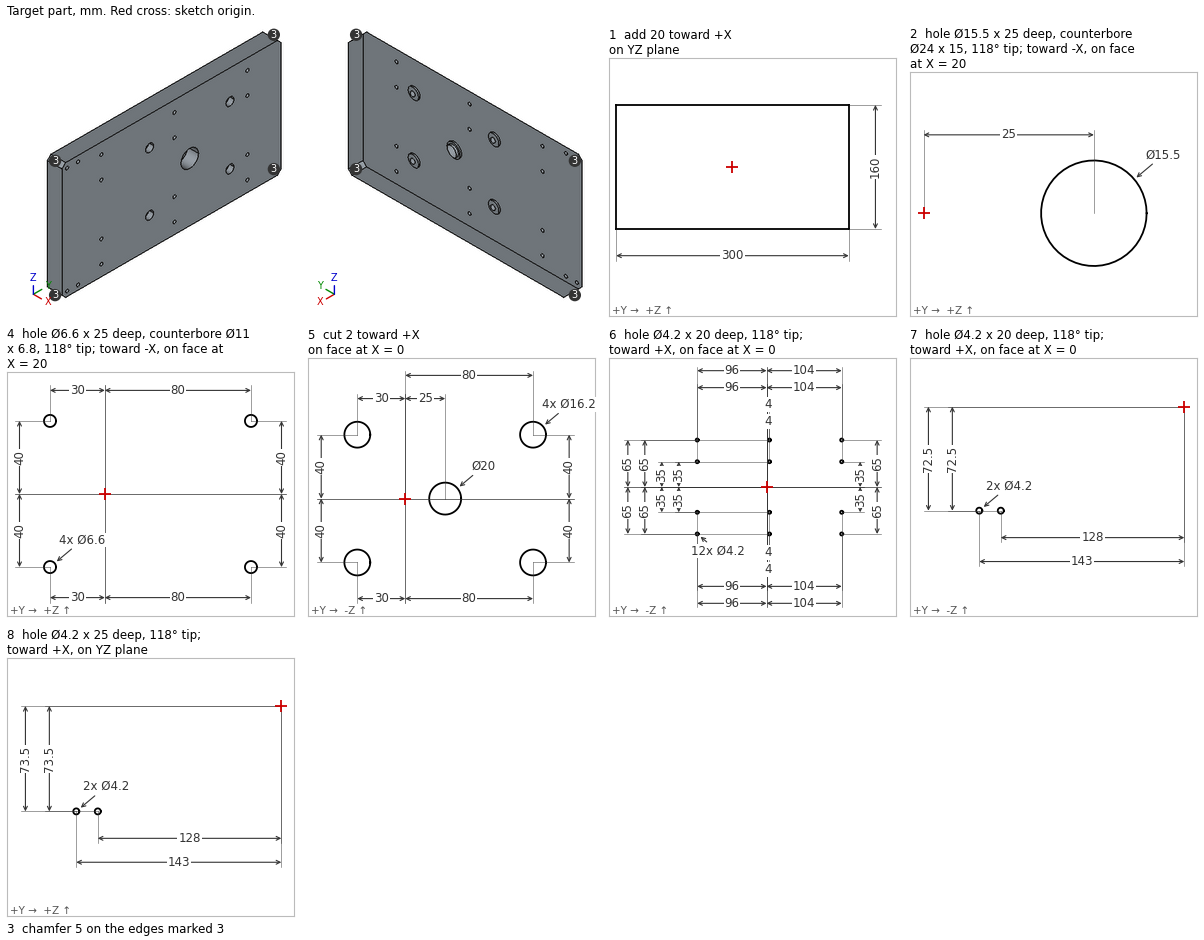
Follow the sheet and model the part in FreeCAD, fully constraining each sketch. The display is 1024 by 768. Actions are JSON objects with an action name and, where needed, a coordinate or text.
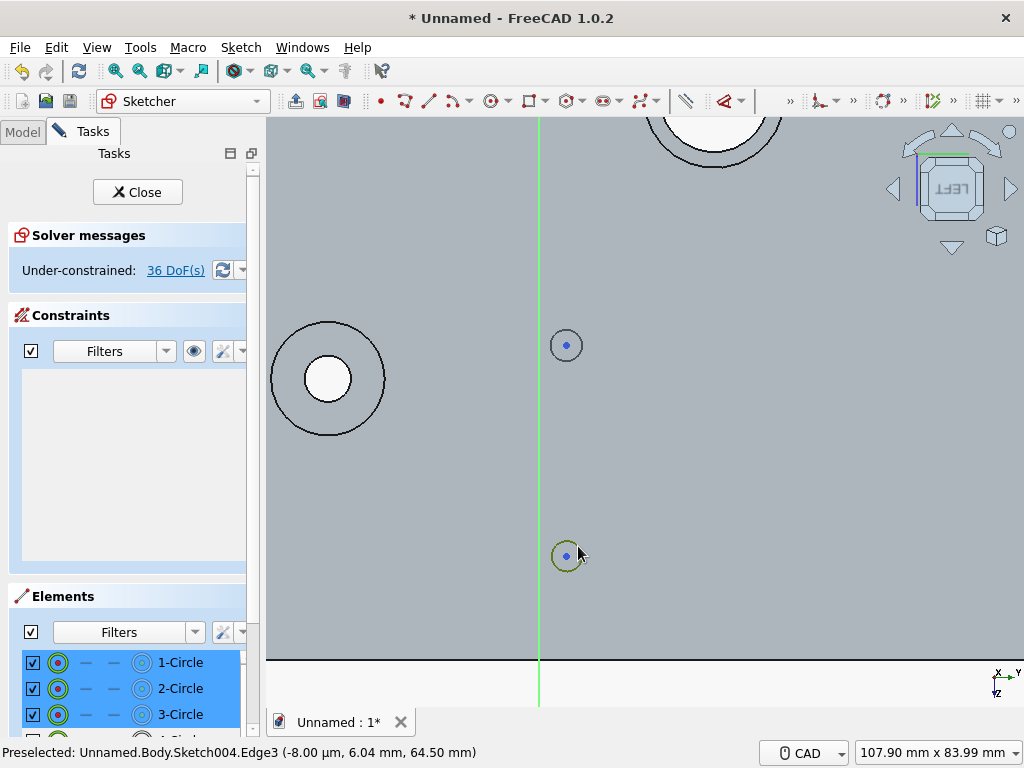
{"action": "left_click", "coordinate": [577, 334]}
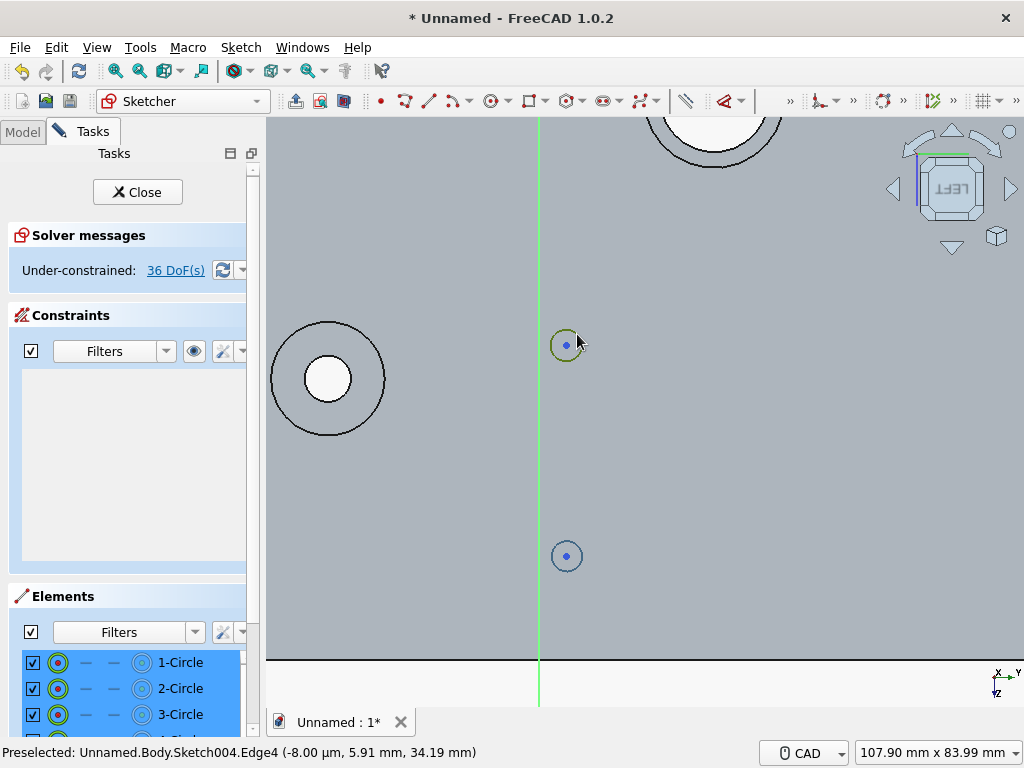
{"action": "scroll", "coordinate": [581, 547], "scroll_direction": "down", "scroll_amount": 6}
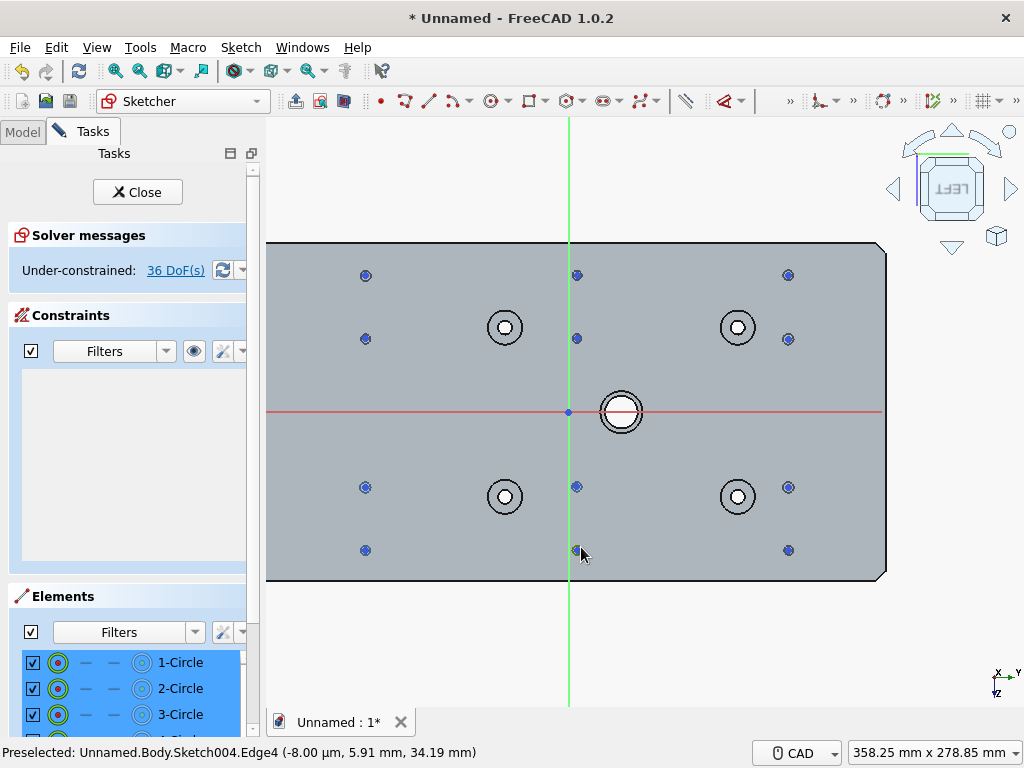
{"action": "scroll", "coordinate": [792, 547], "scroll_direction": "up", "scroll_amount": 6}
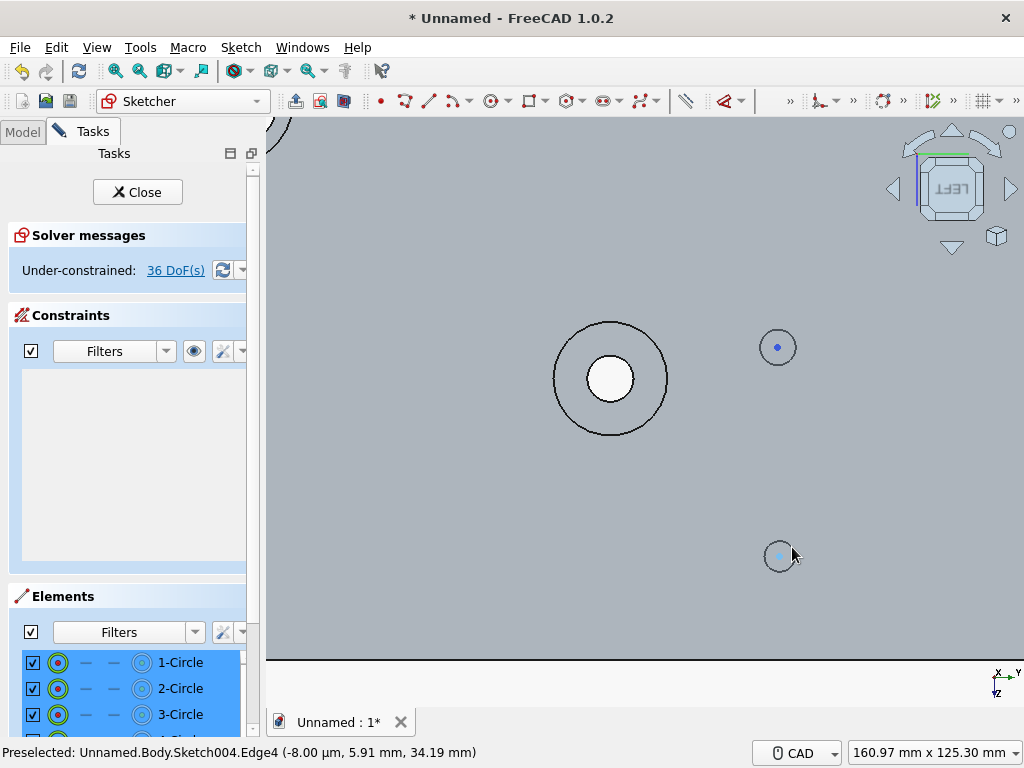
{"action": "left_click", "coordinate": [790, 546]}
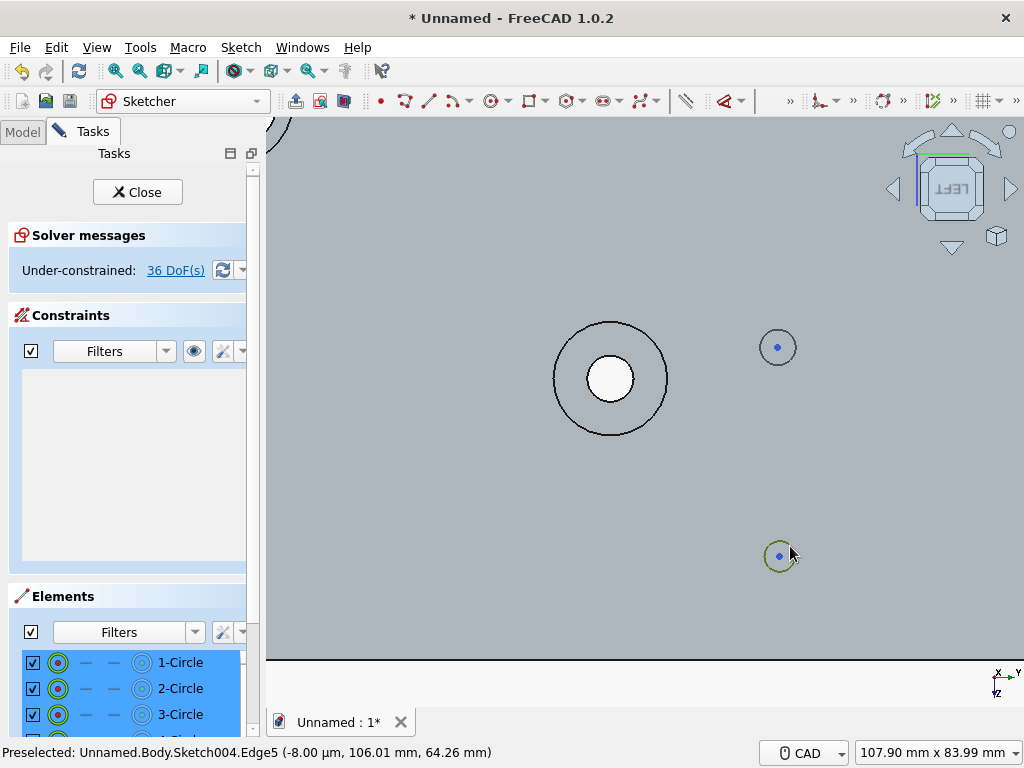
{"action": "left_click", "coordinate": [790, 335]}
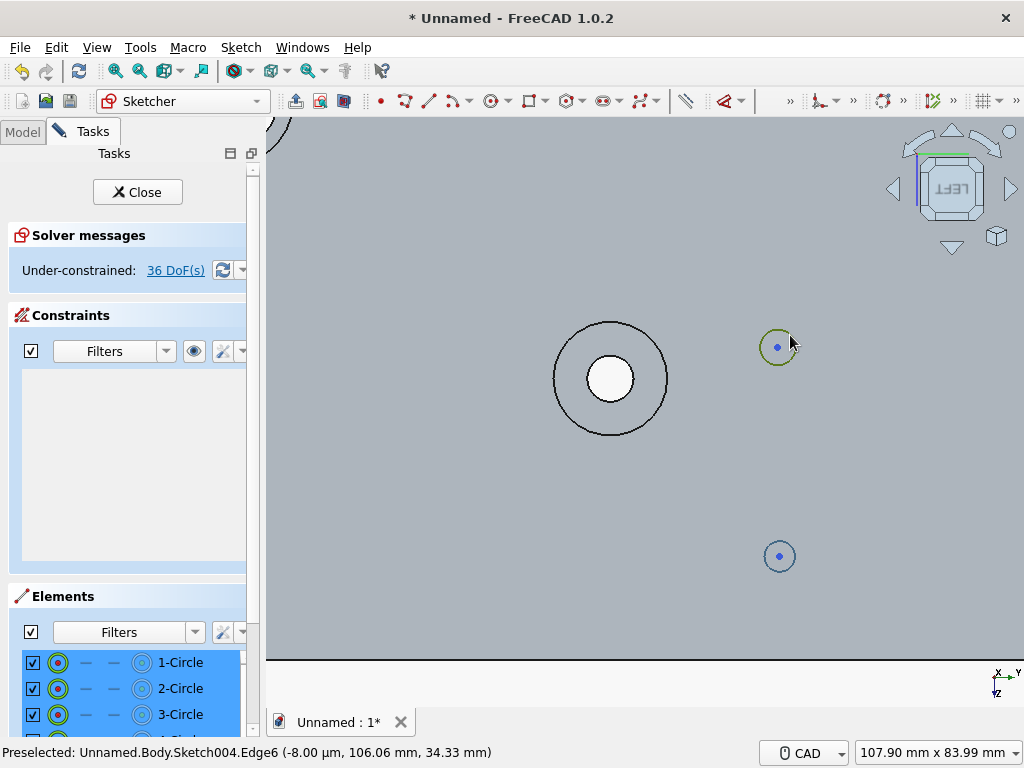
{"action": "scroll", "coordinate": [792, 547], "scroll_direction": "down", "scroll_amount": 6}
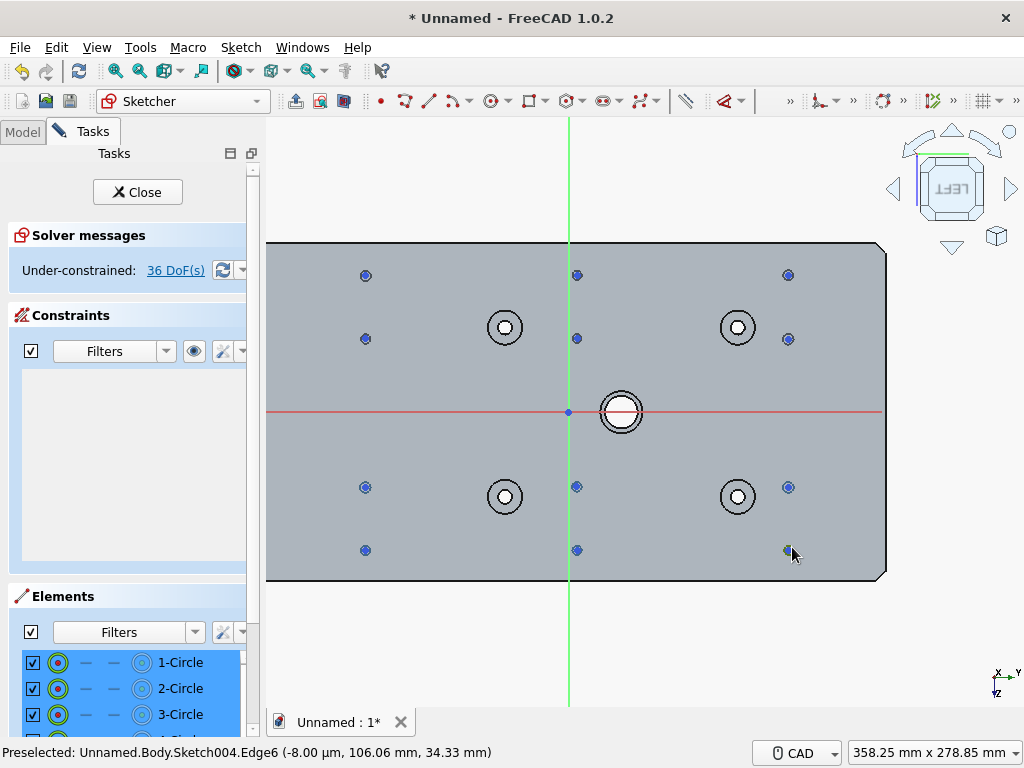
{"action": "scroll", "coordinate": [792, 335], "scroll_direction": "up", "scroll_amount": 5}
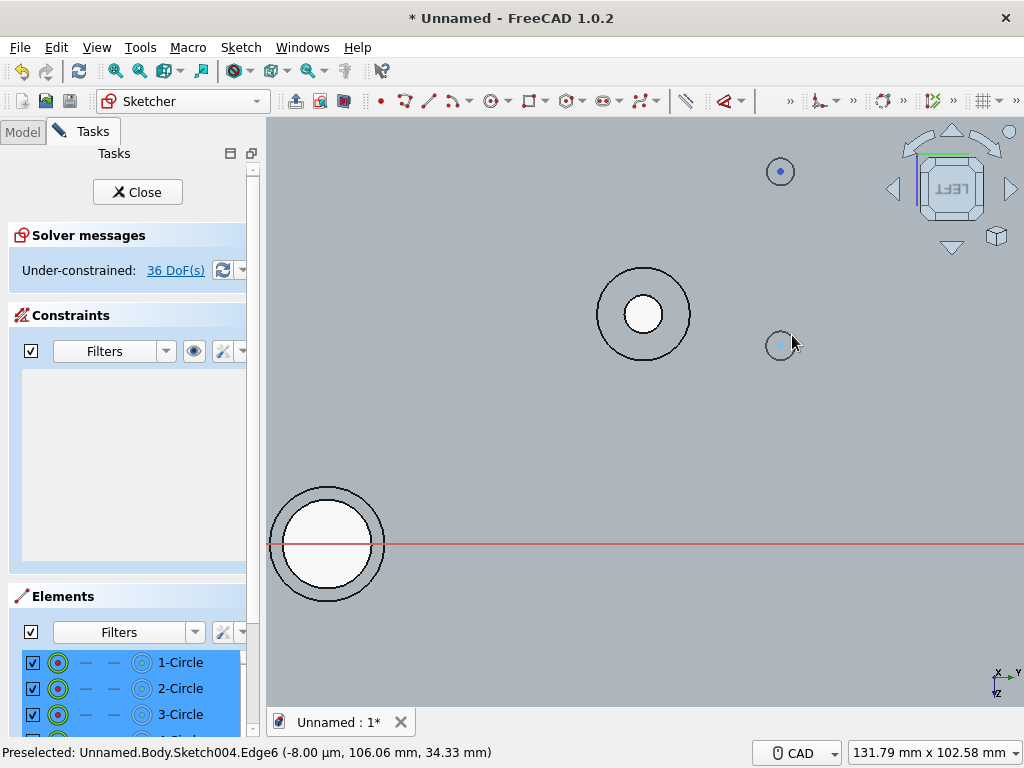
{"action": "left_click", "coordinate": [791, 336]}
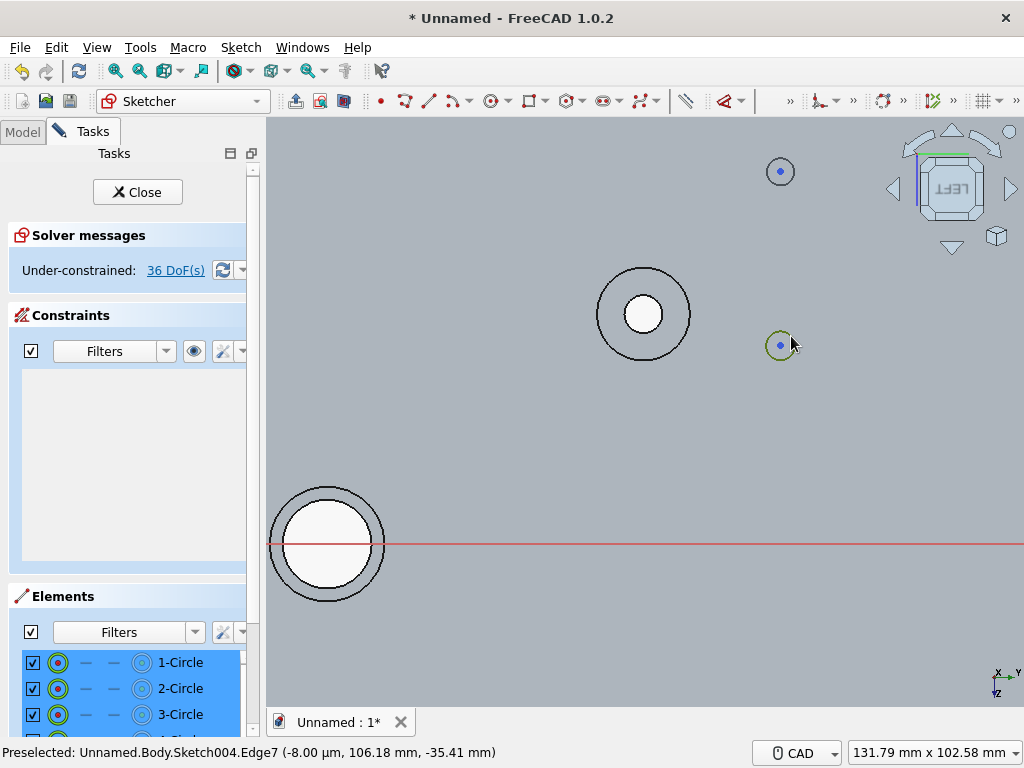
{"action": "left_click", "coordinate": [790, 162]}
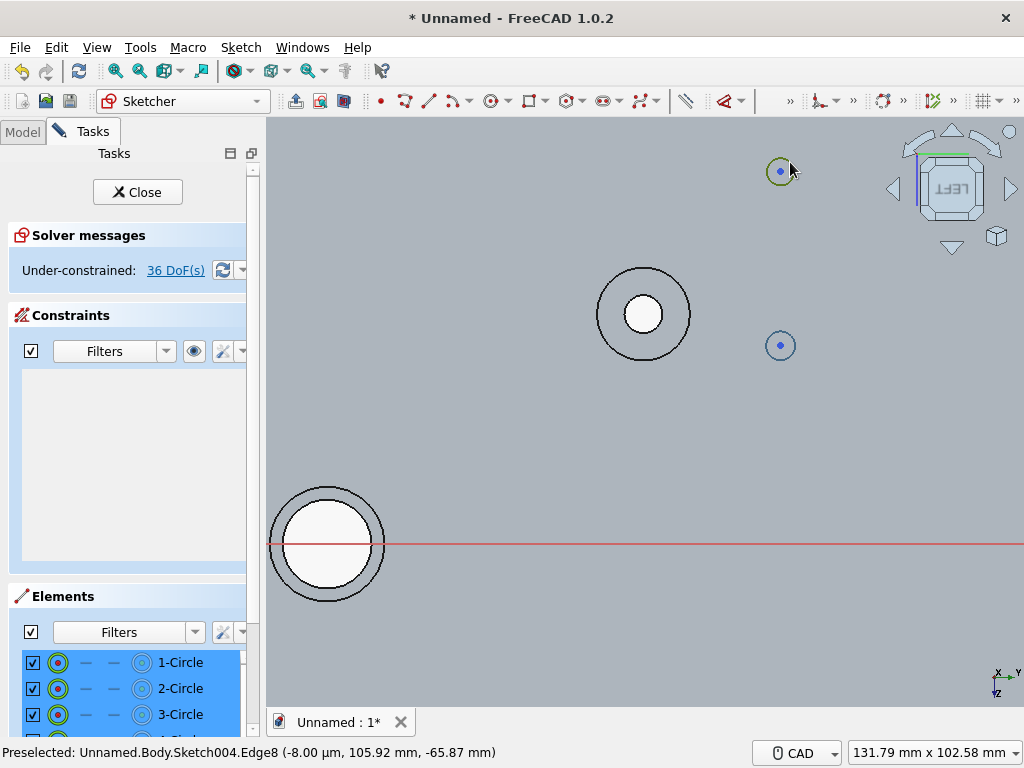
{"action": "scroll", "coordinate": [792, 335], "scroll_direction": "down", "scroll_amount": 5}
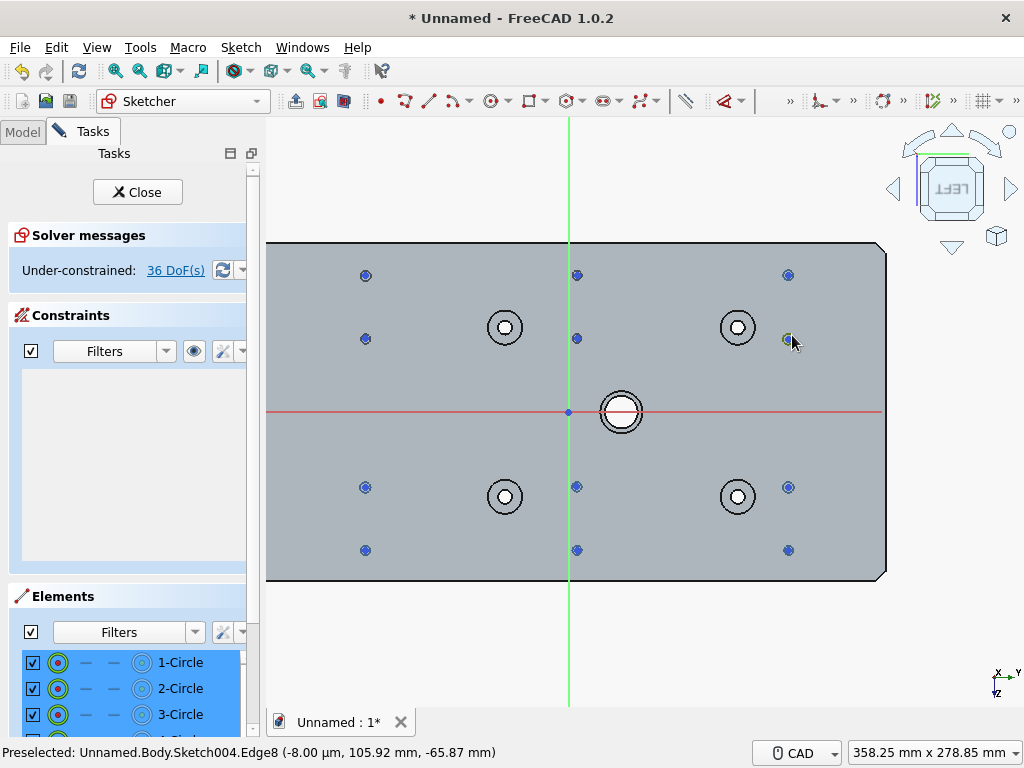
{"action": "scroll", "coordinate": [580, 335], "scroll_direction": "up", "scroll_amount": 6}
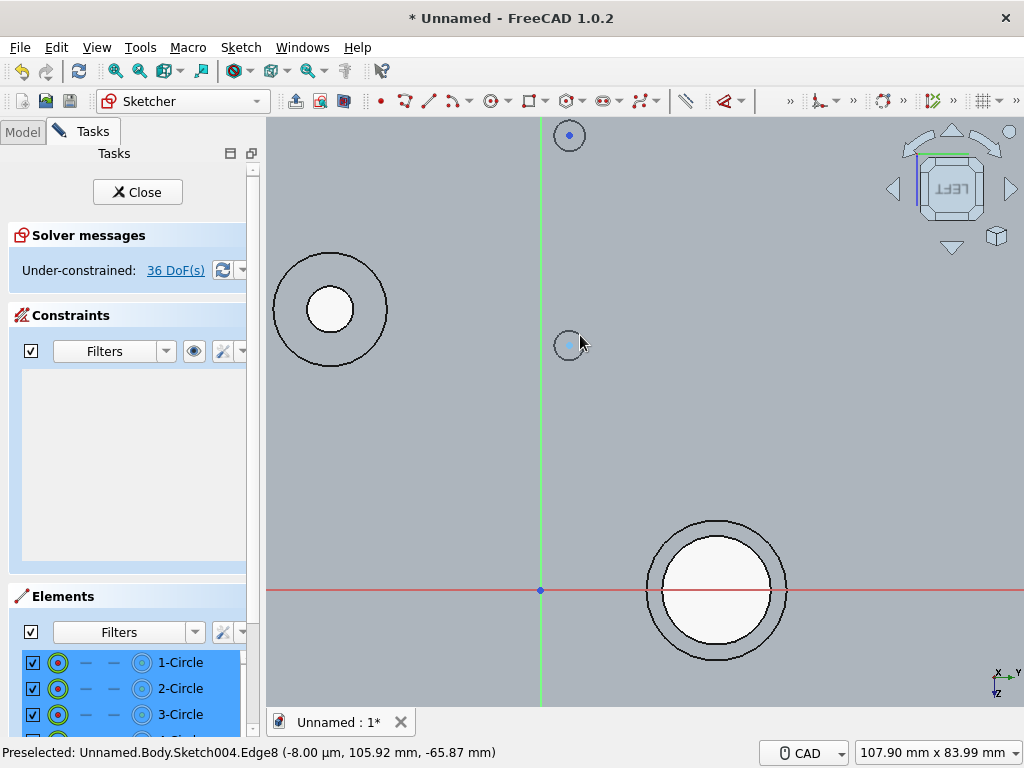
{"action": "left_click", "coordinate": [580, 335]}